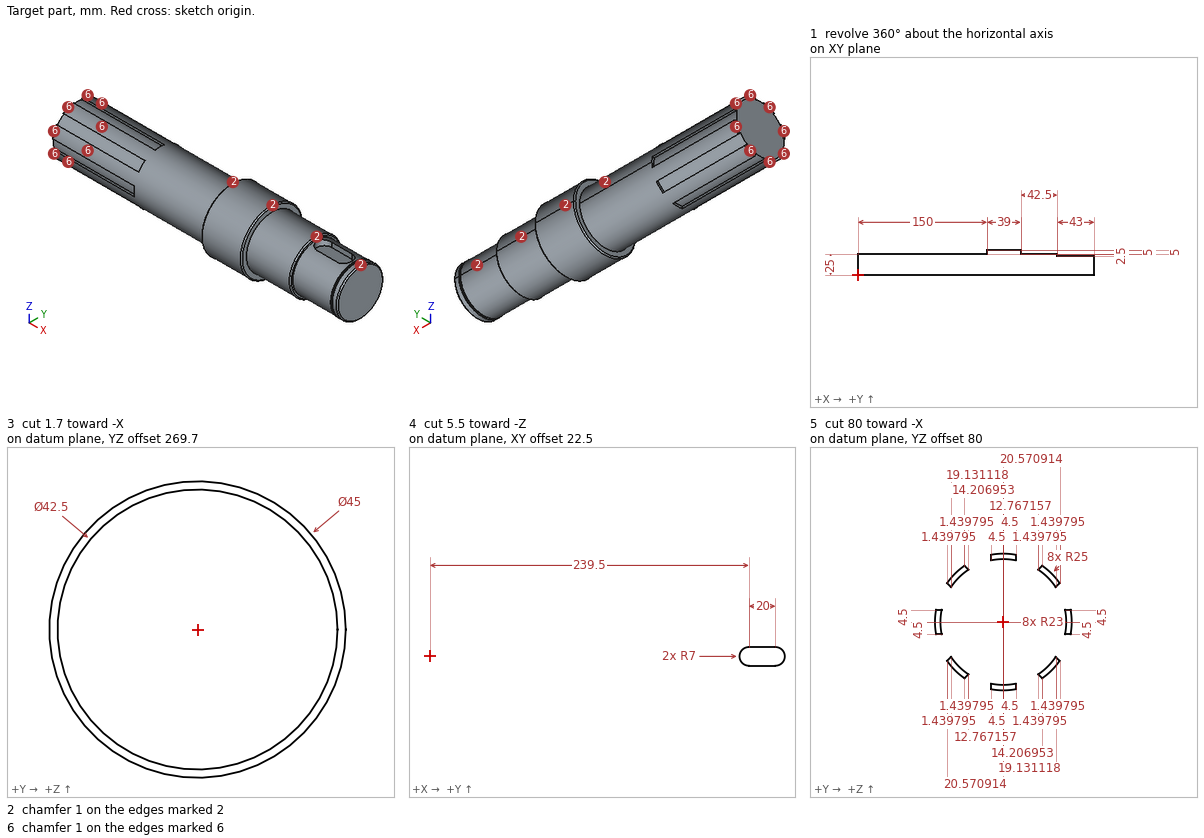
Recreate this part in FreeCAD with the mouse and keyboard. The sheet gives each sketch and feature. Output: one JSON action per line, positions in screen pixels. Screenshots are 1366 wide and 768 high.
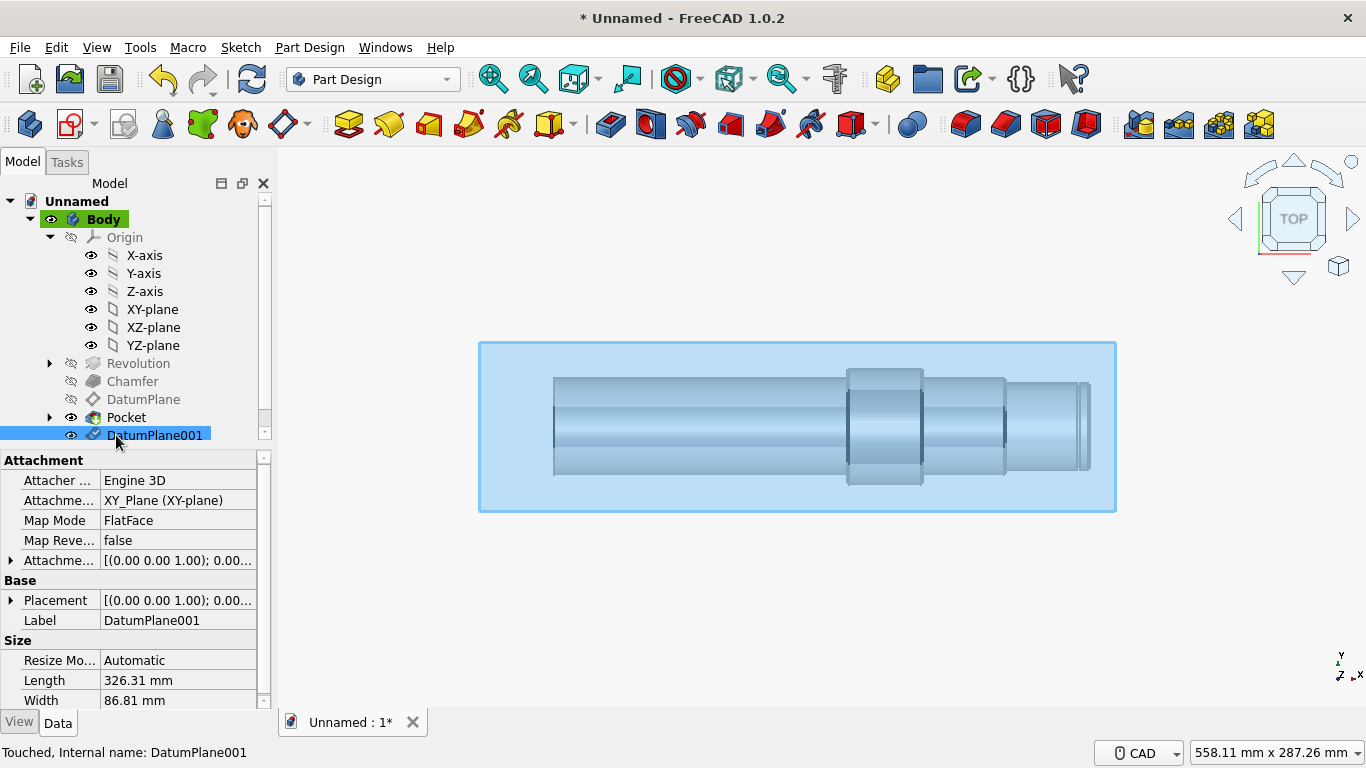
{"action": "left_click", "coordinate": [70, 124]}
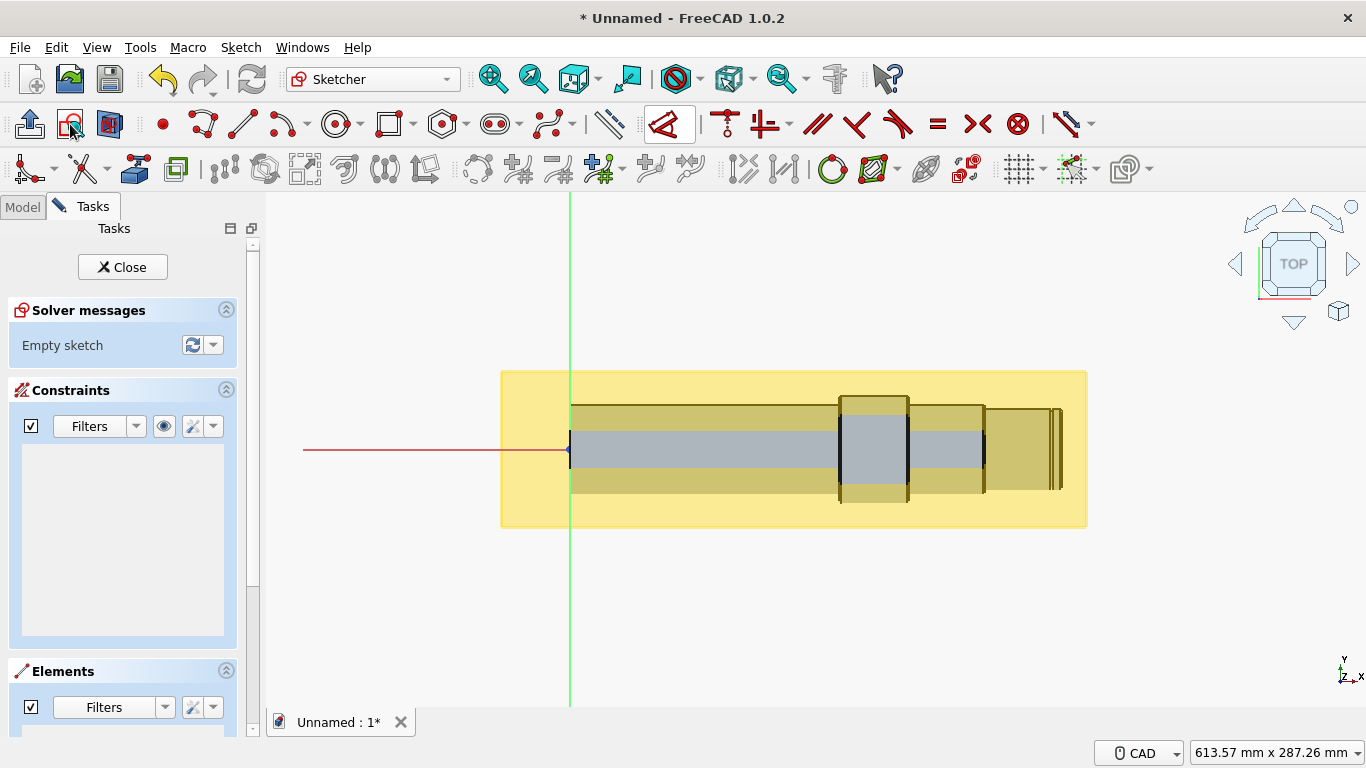
{"action": "left_click", "coordinate": [110, 124]}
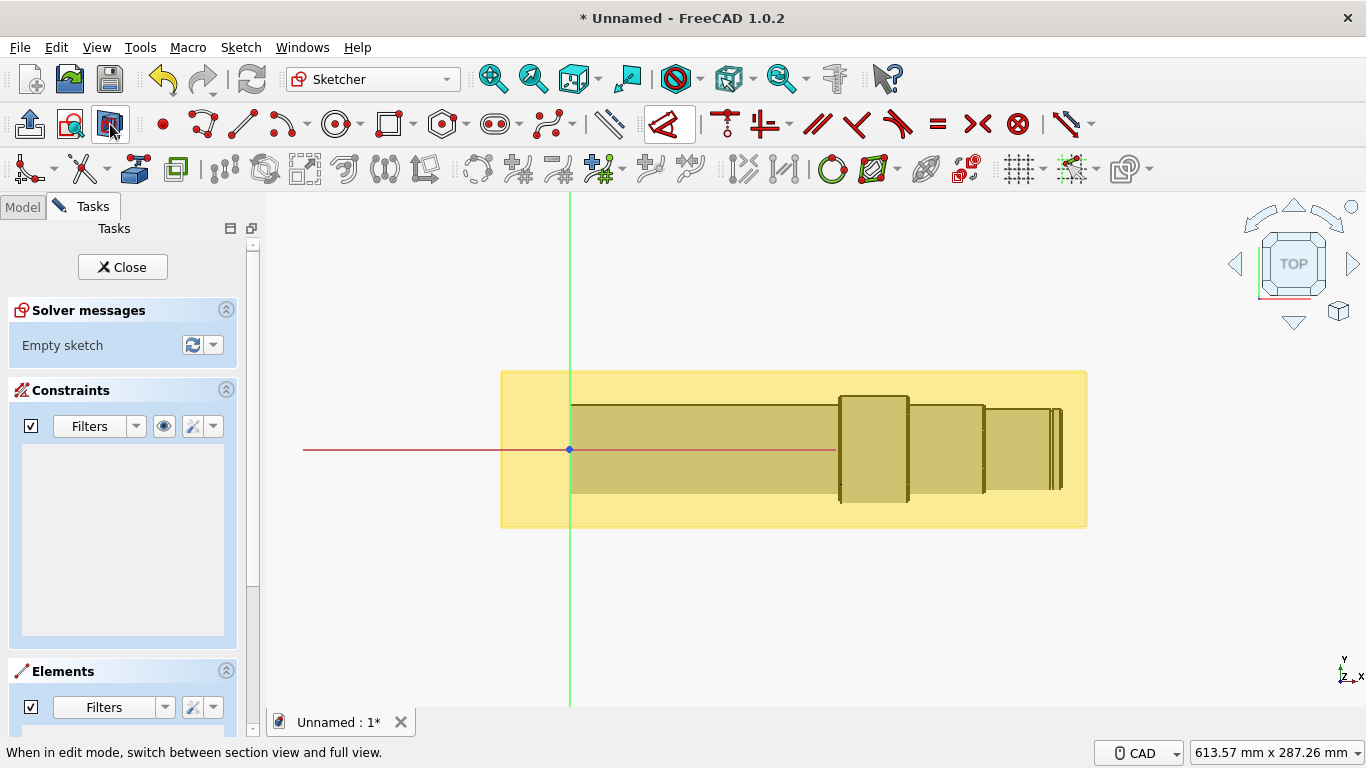
{"action": "scroll", "coordinate": [1044, 450], "scroll_direction": "up", "scroll_amount": 12}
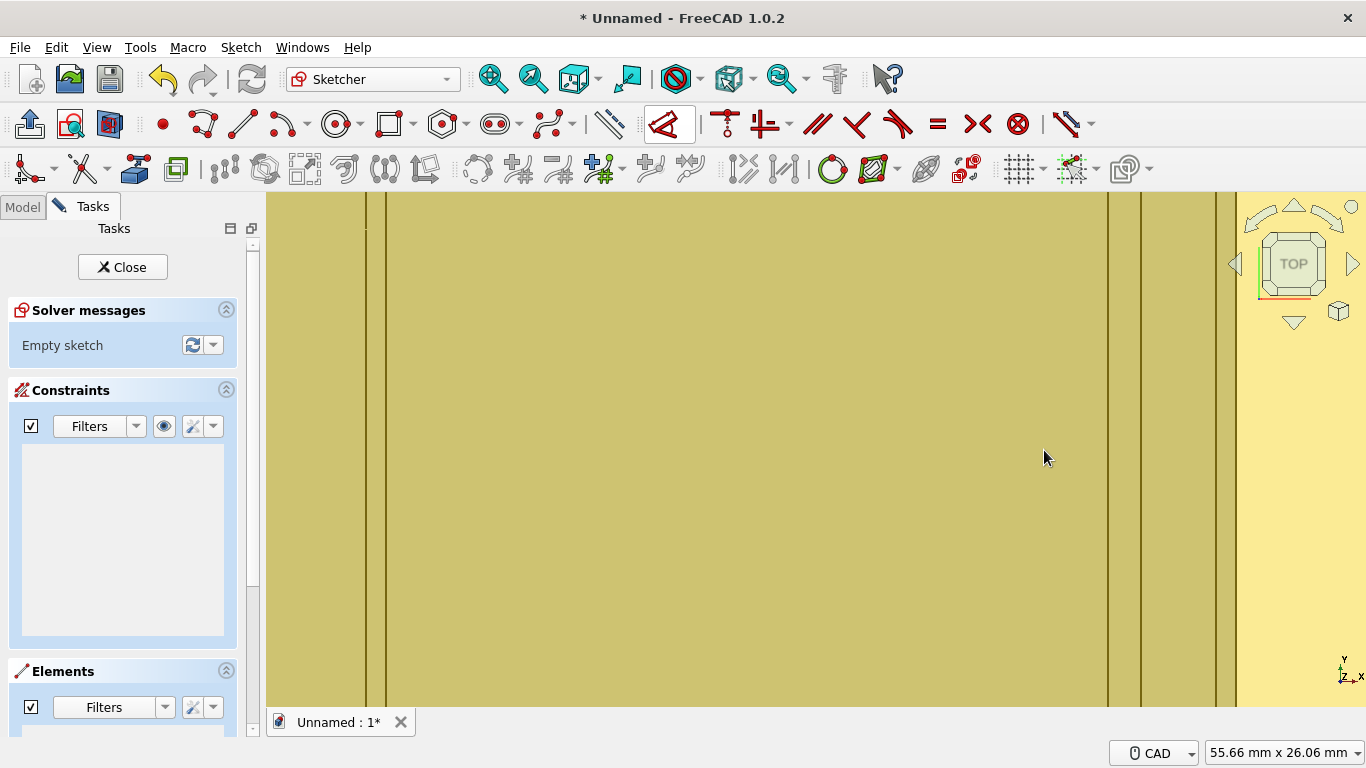
{"action": "left_click", "coordinate": [496, 124]}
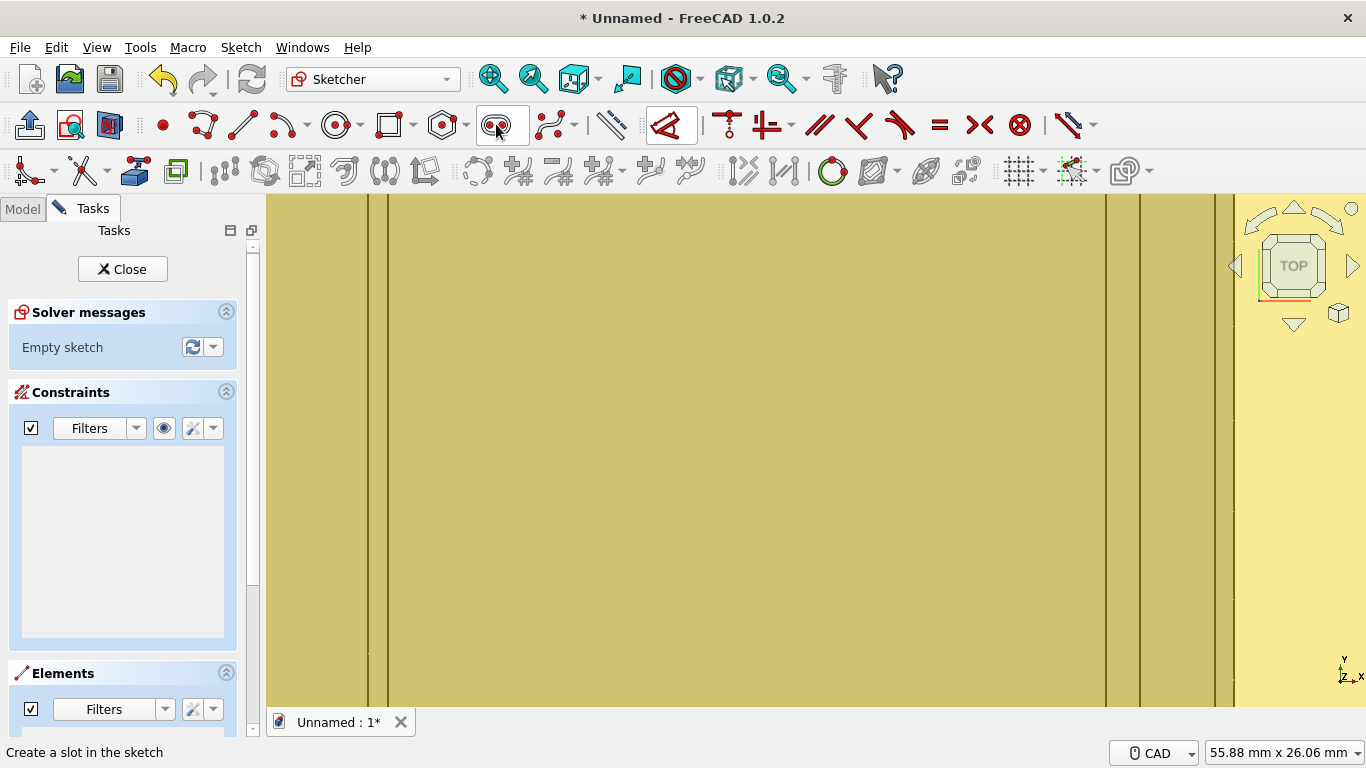
{"action": "left_click", "coordinate": [545, 440]}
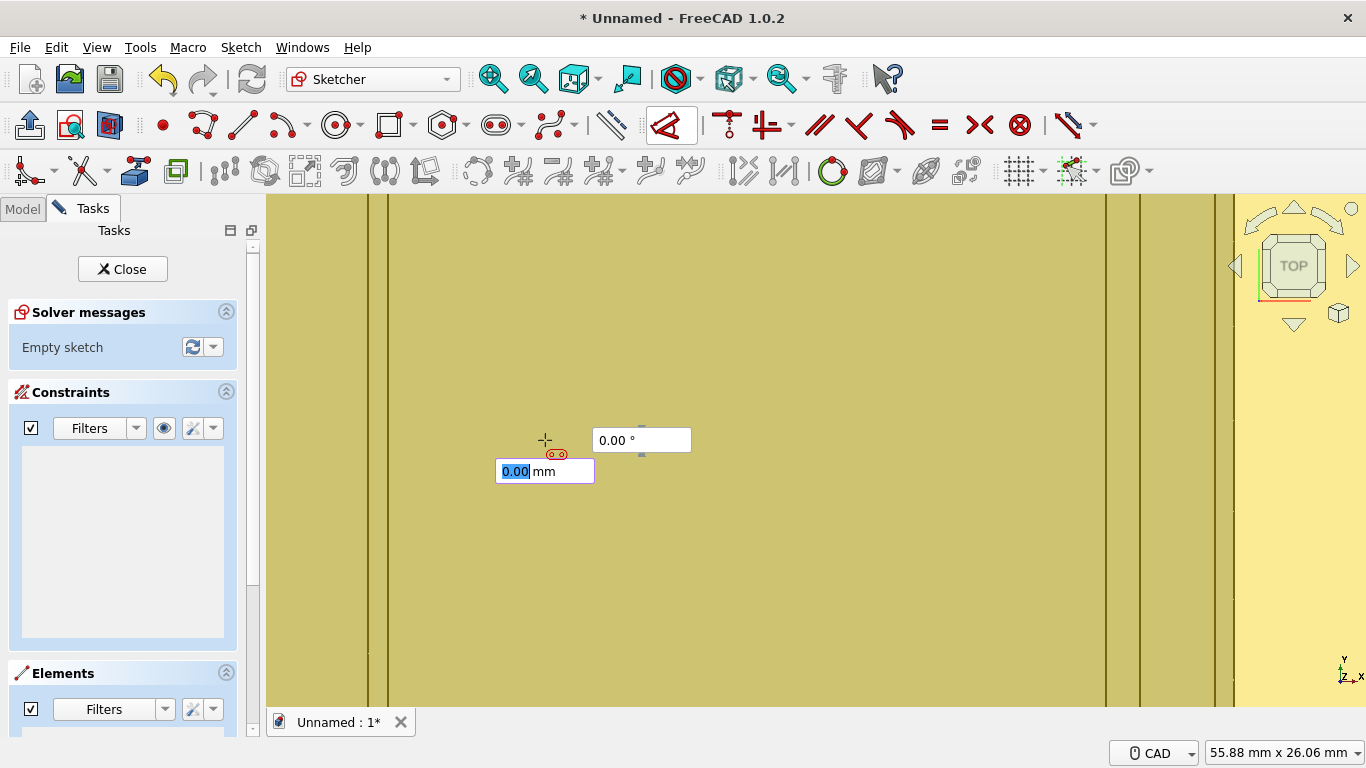
{"action": "left_click", "coordinate": [939, 431]}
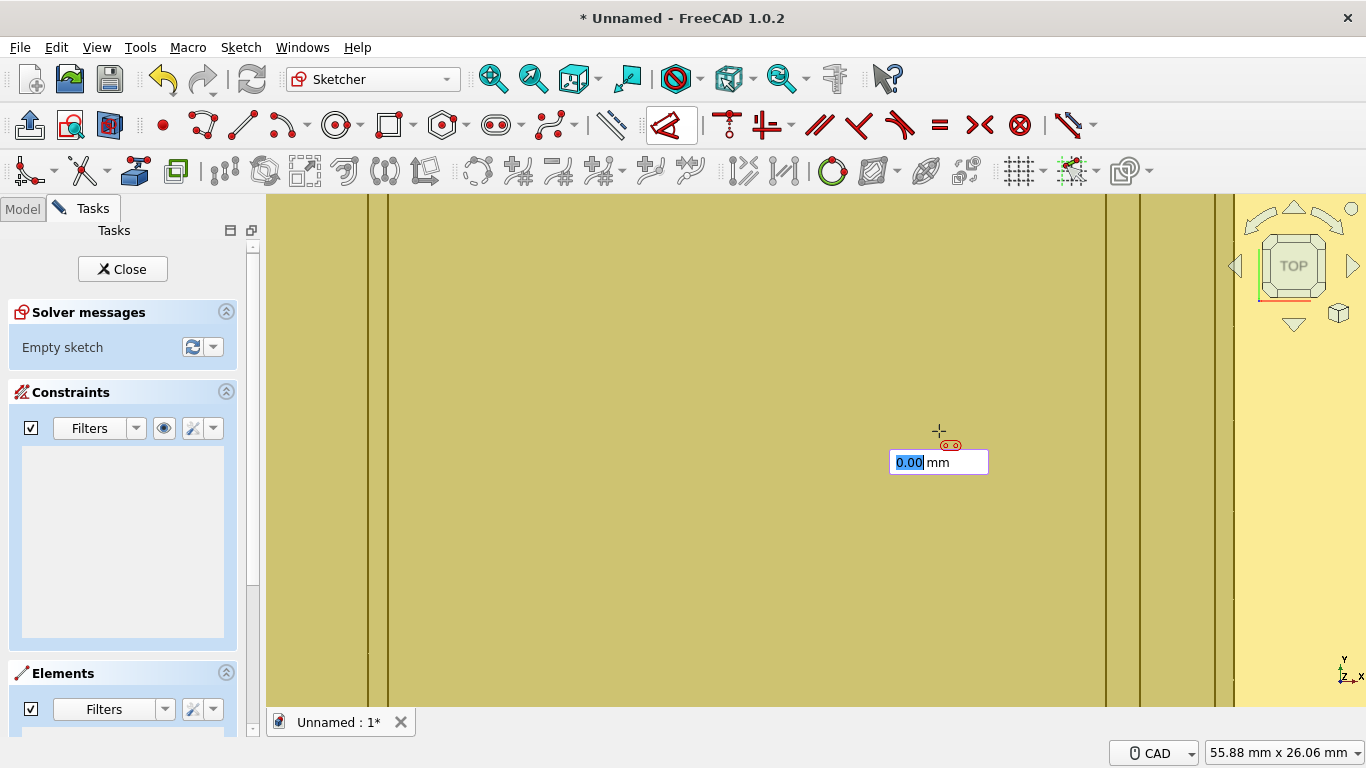
{"action": "left_click", "coordinate": [742, 303]}
{"action": "key", "text": "Escape"}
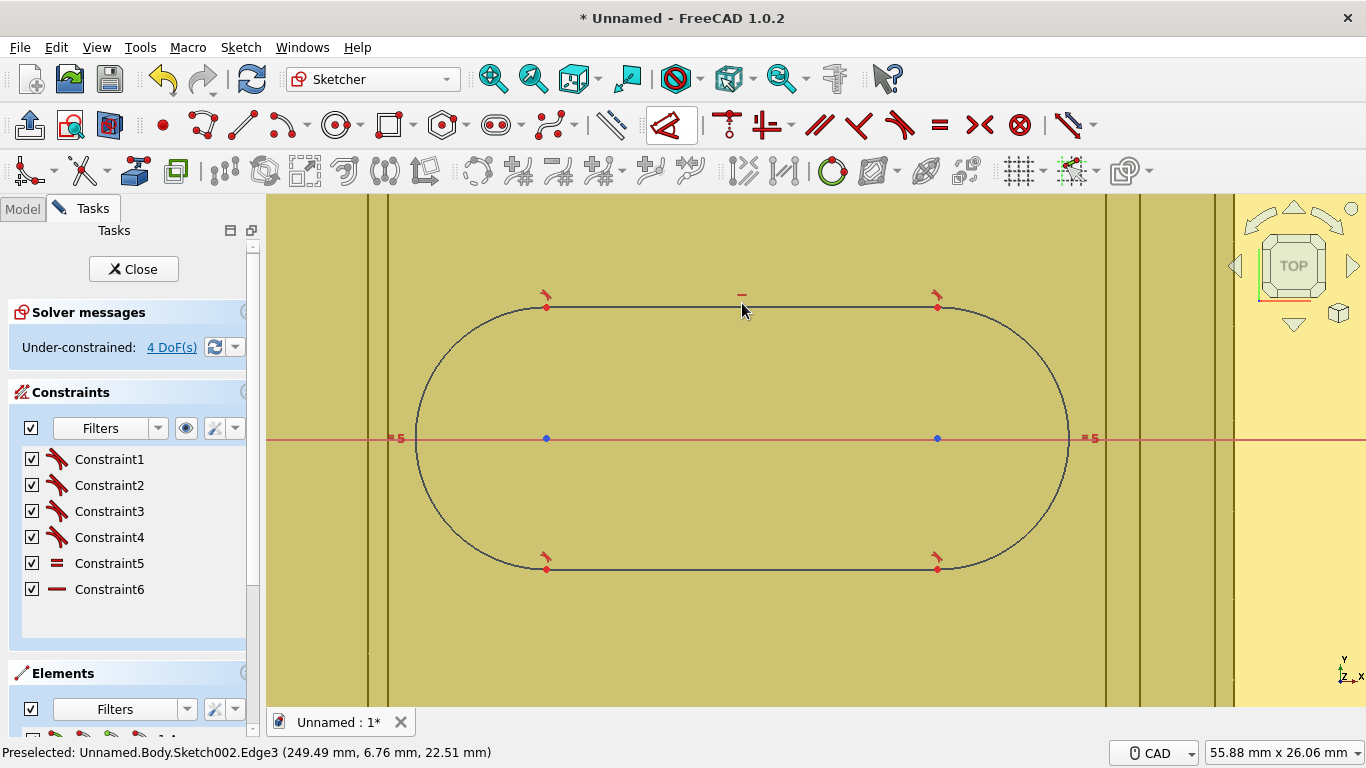
{"action": "left_click", "coordinate": [547, 438]}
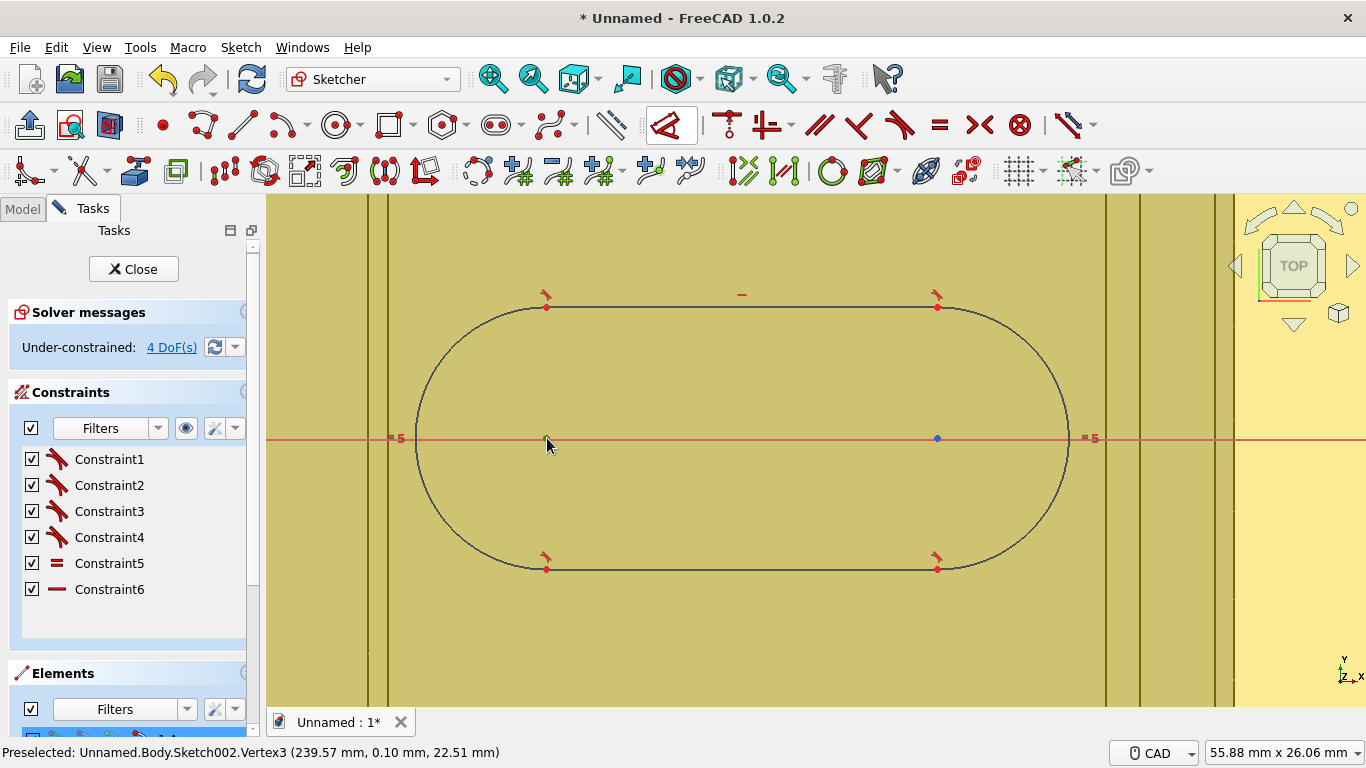
{"action": "left_click", "coordinate": [359, 440]}